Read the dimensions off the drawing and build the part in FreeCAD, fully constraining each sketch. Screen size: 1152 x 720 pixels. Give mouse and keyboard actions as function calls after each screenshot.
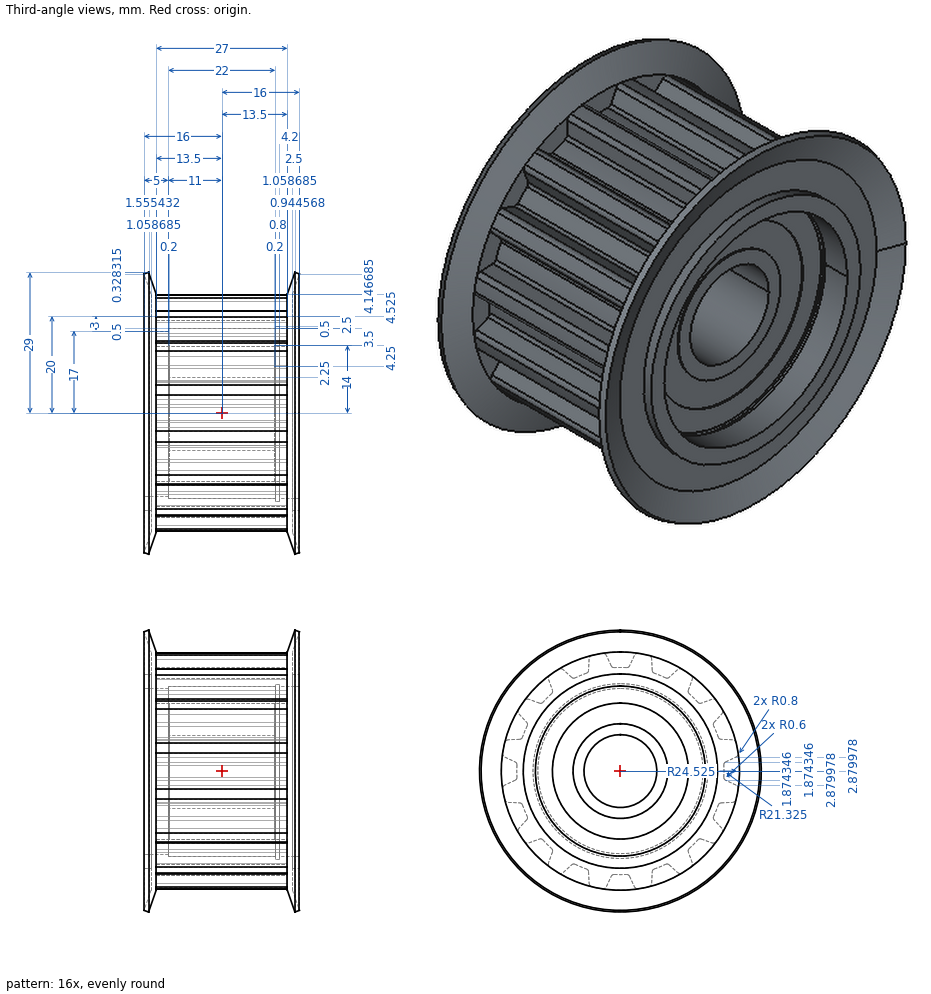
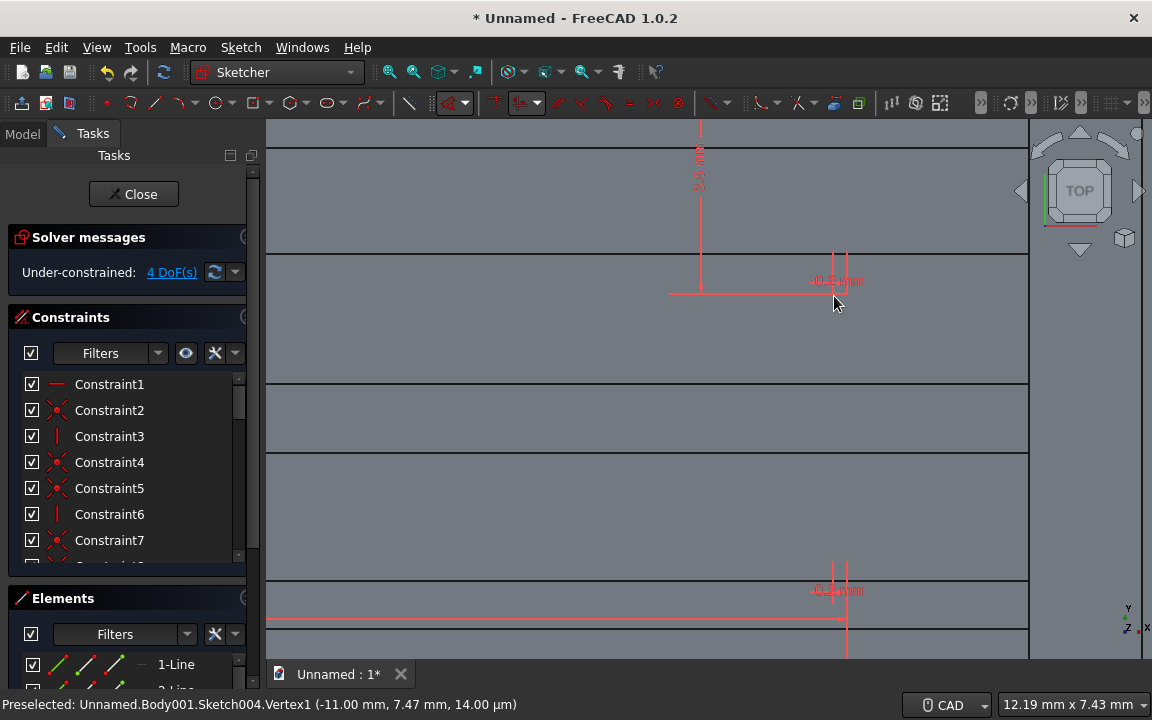
click(833, 294)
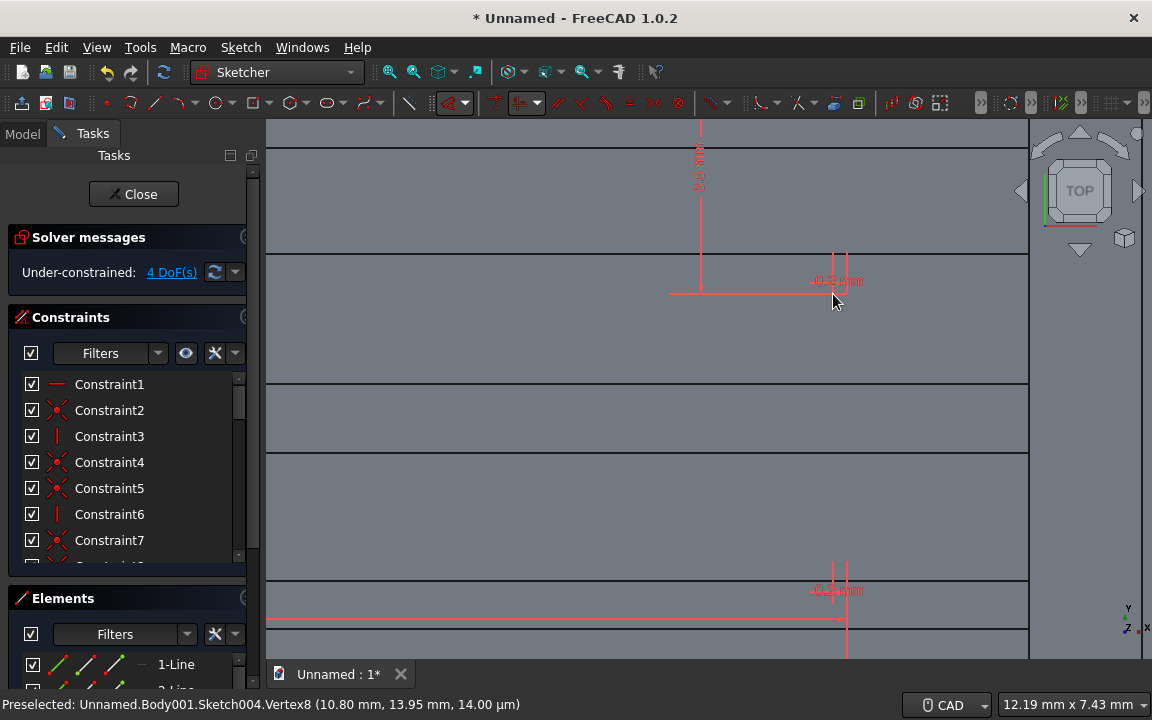
click(468, 104)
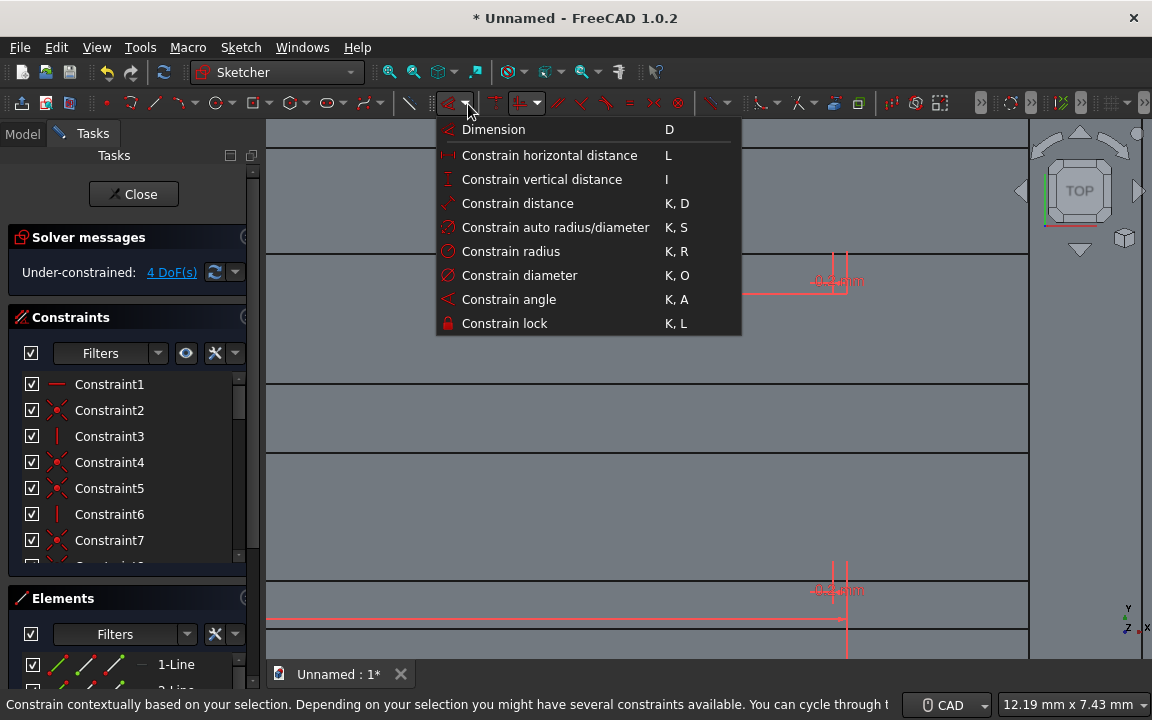
click(589, 179)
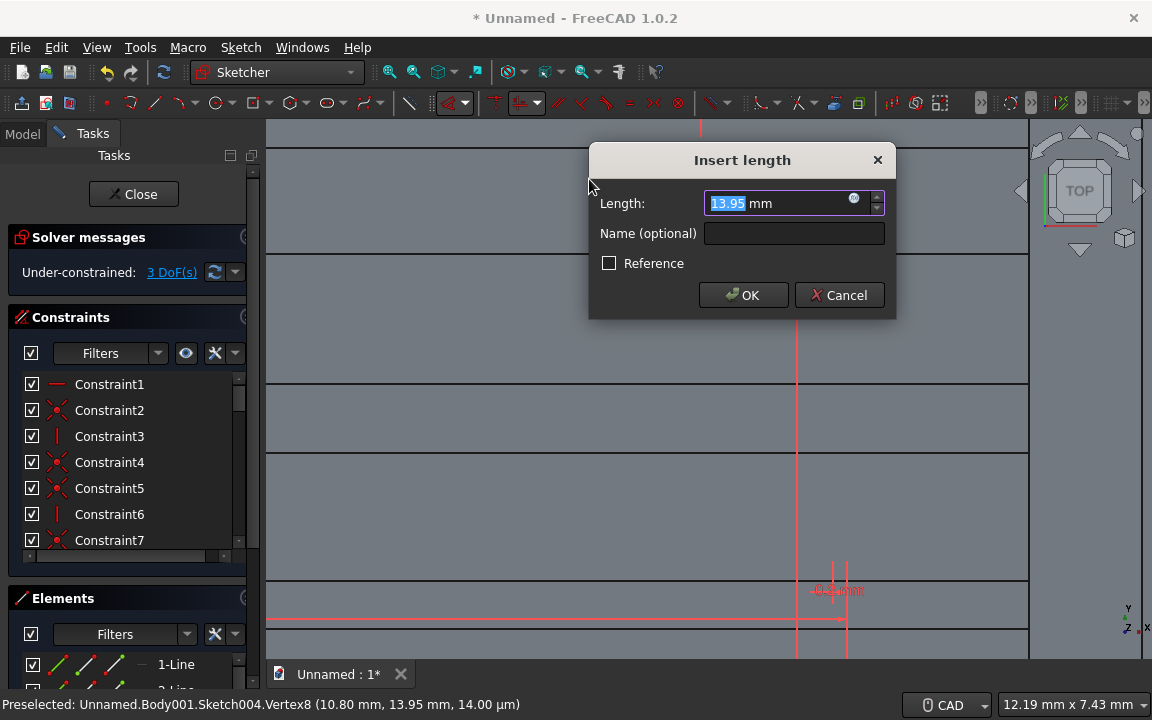
text(14)
key(Return)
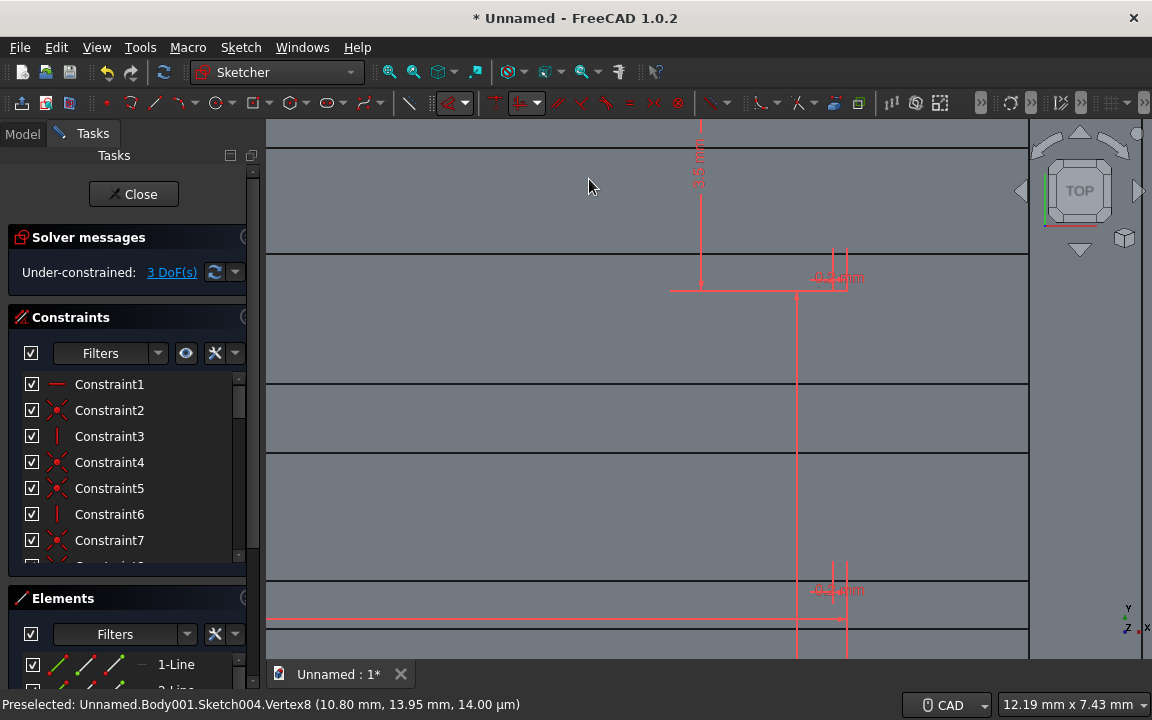
scroll(835, 296, down, 7)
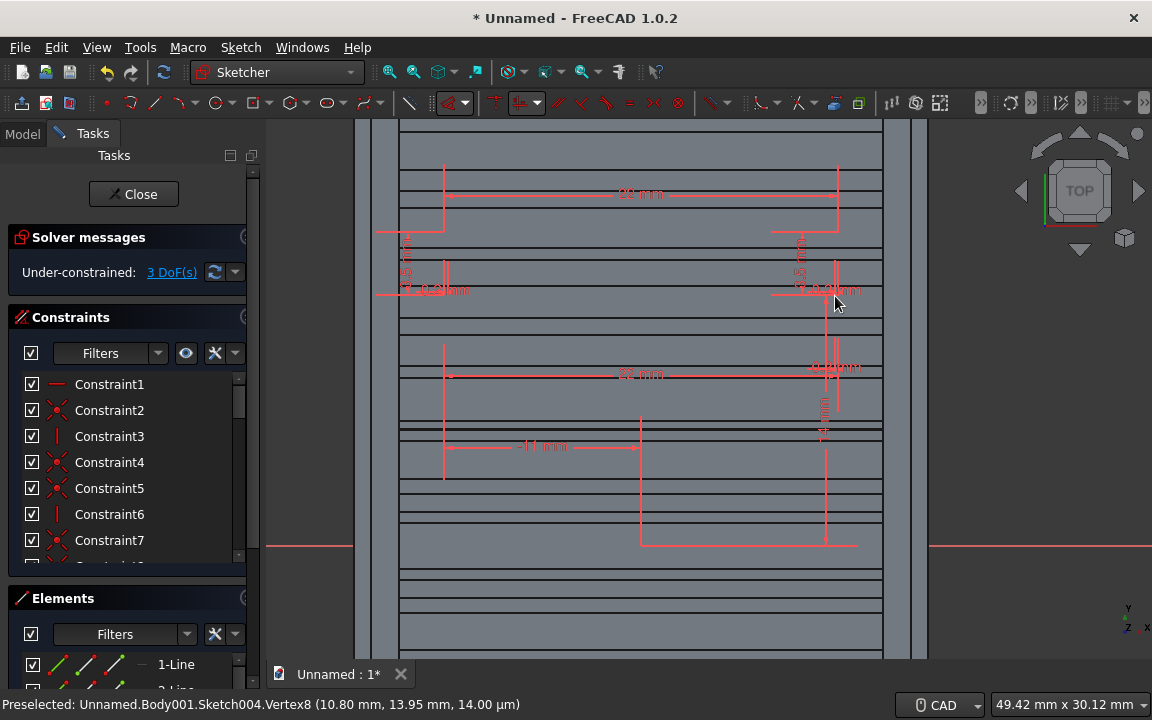
click(838, 400)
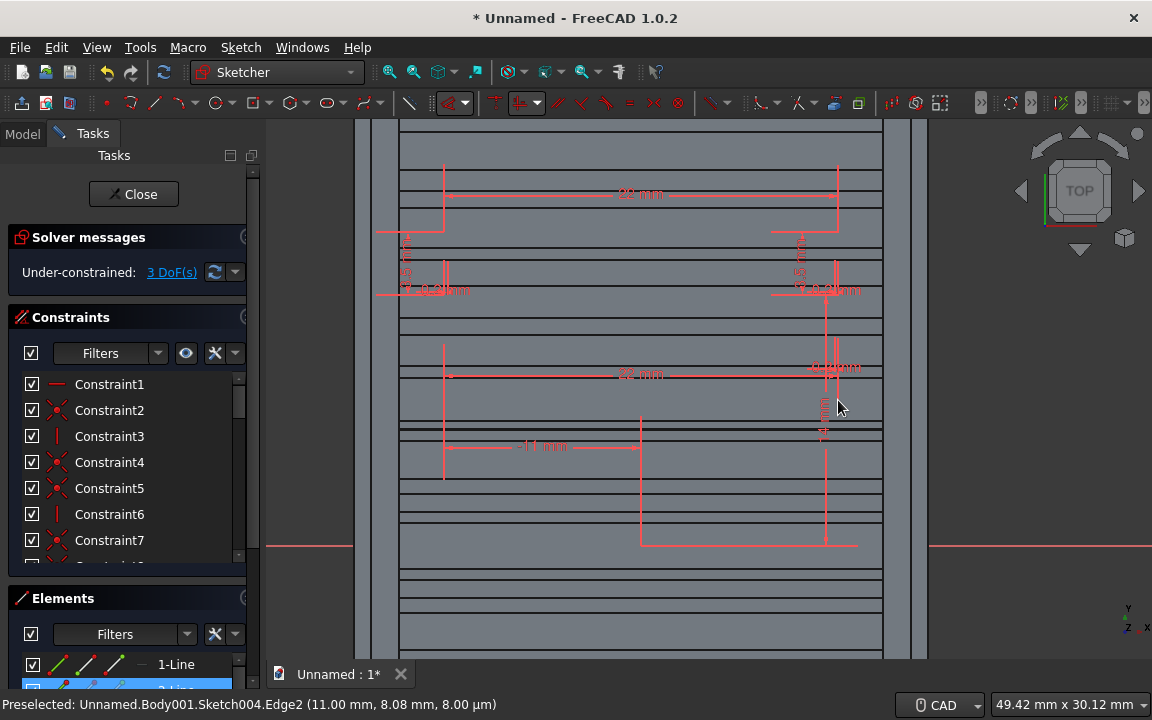
key(i)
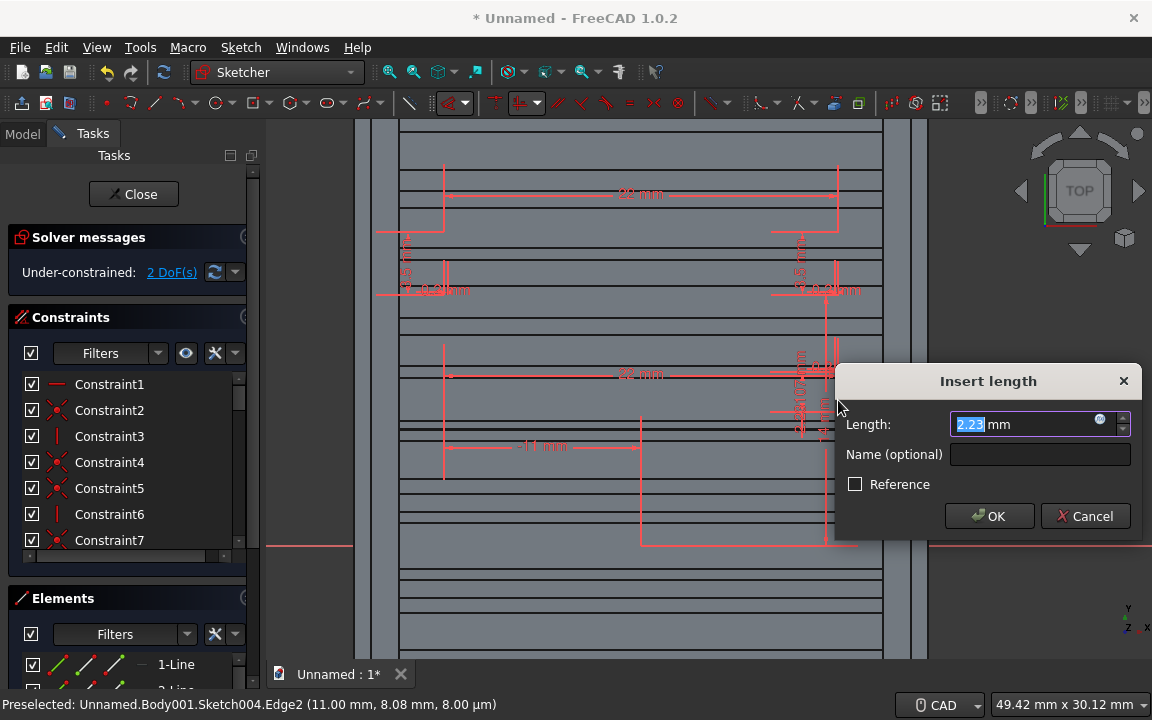
text(2.25)
key(Return)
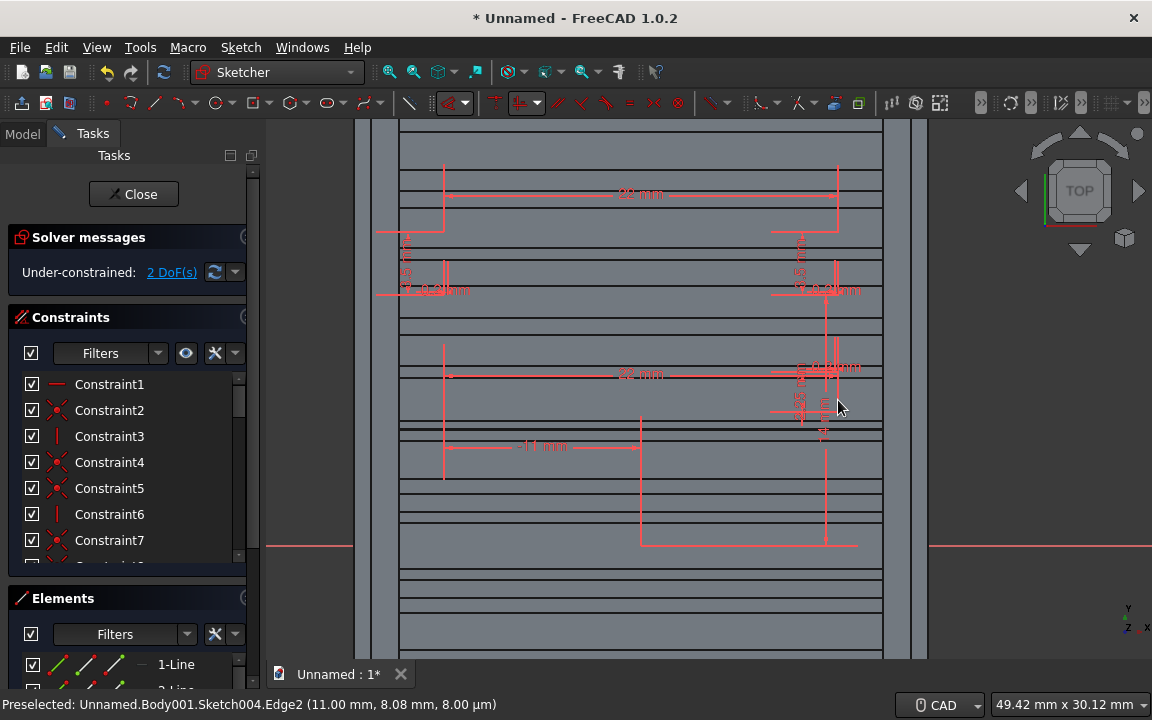
click(835, 349)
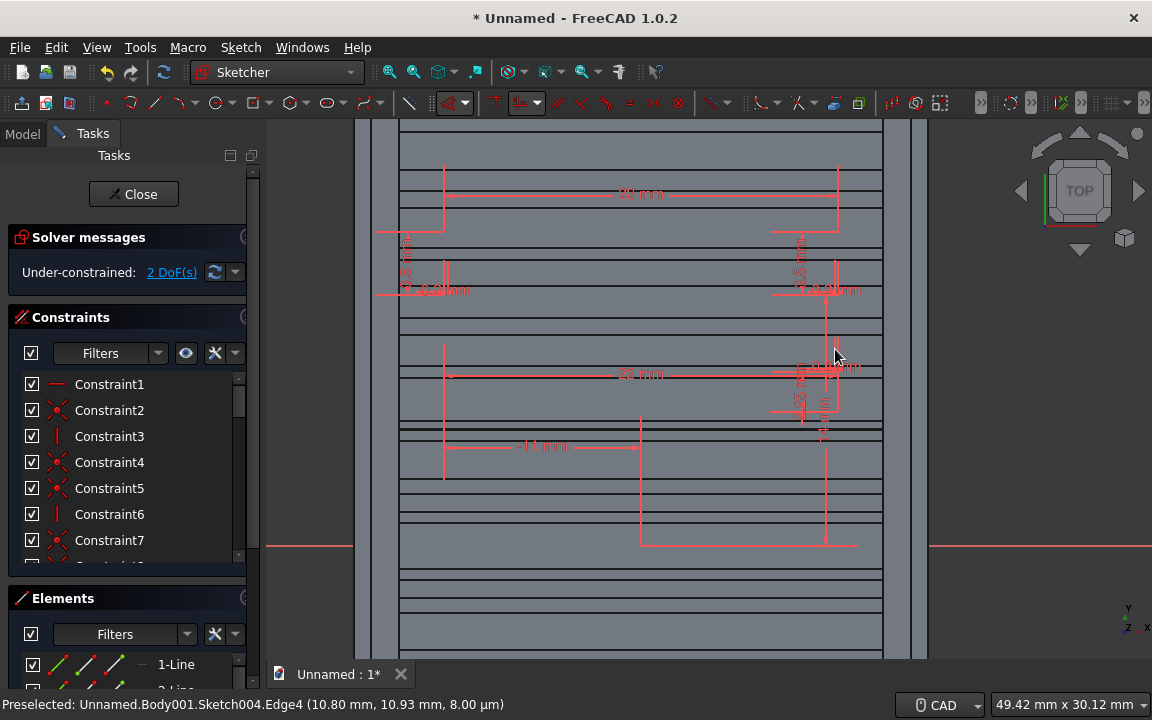
click(468, 104)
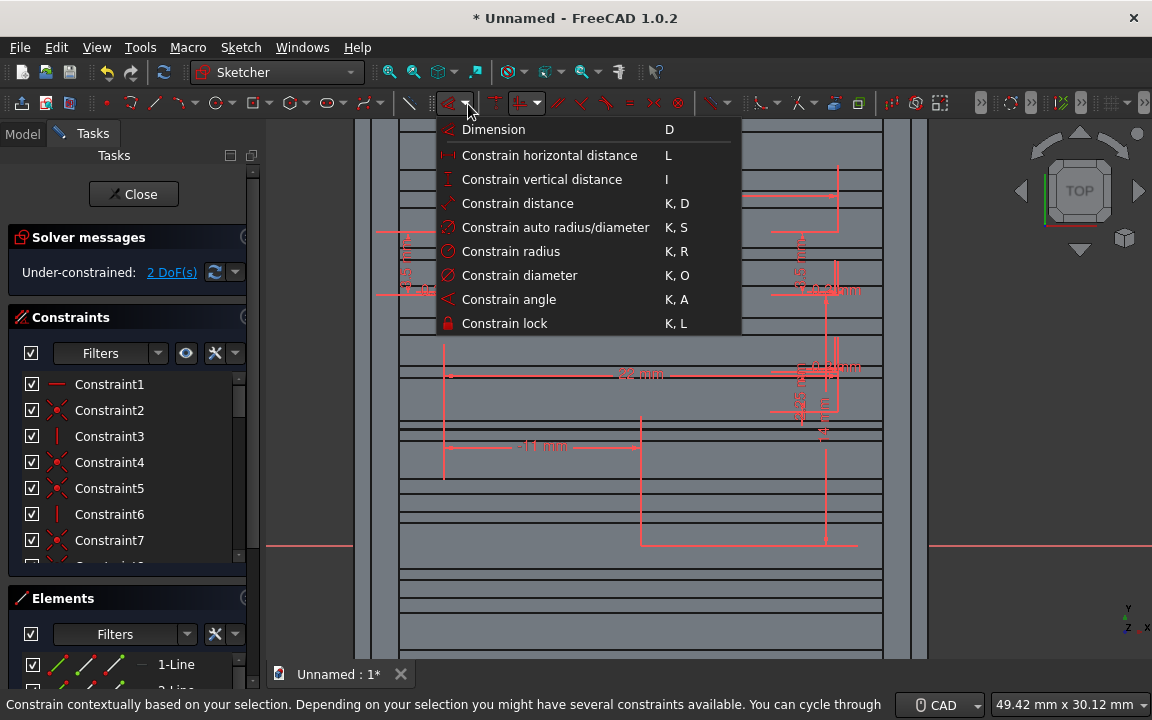
click(589, 179)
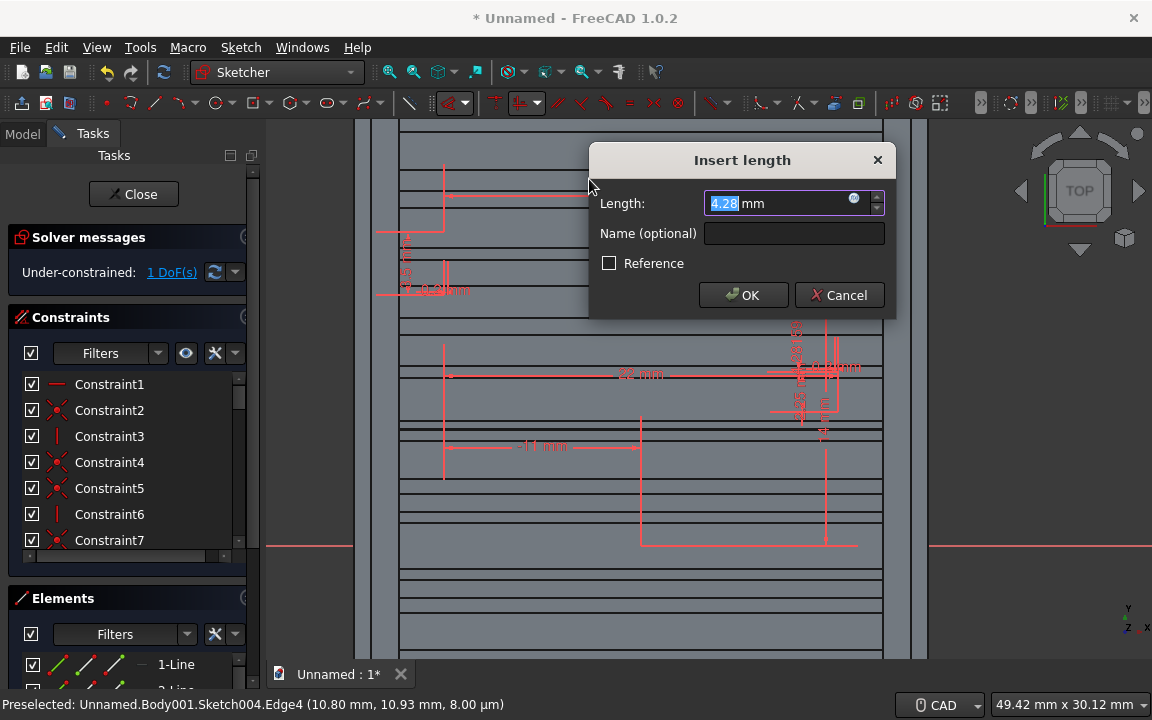
text(4.25)
key(Return)